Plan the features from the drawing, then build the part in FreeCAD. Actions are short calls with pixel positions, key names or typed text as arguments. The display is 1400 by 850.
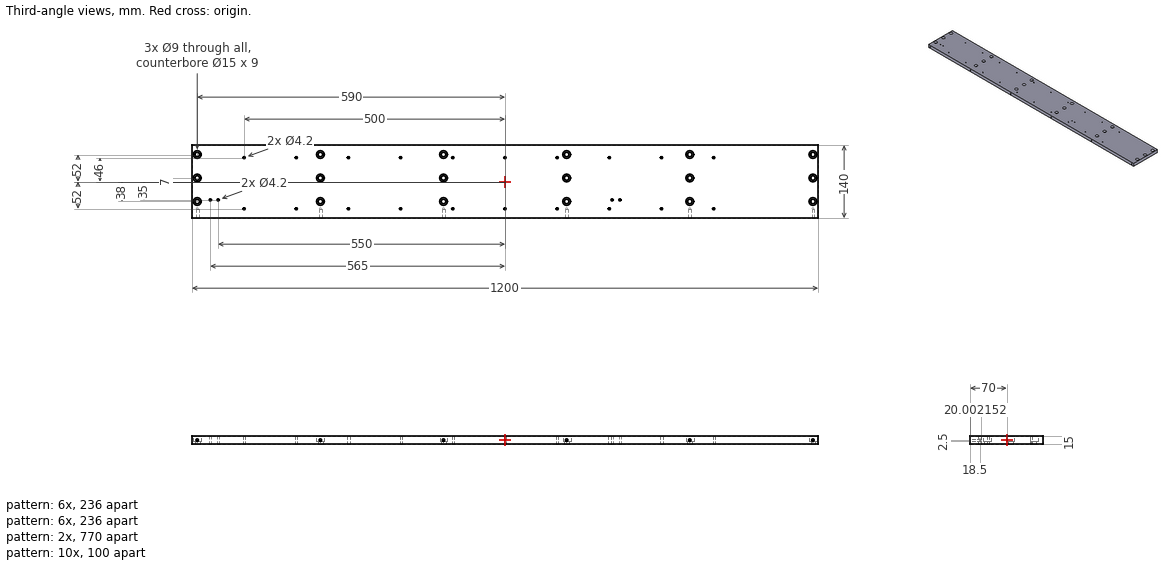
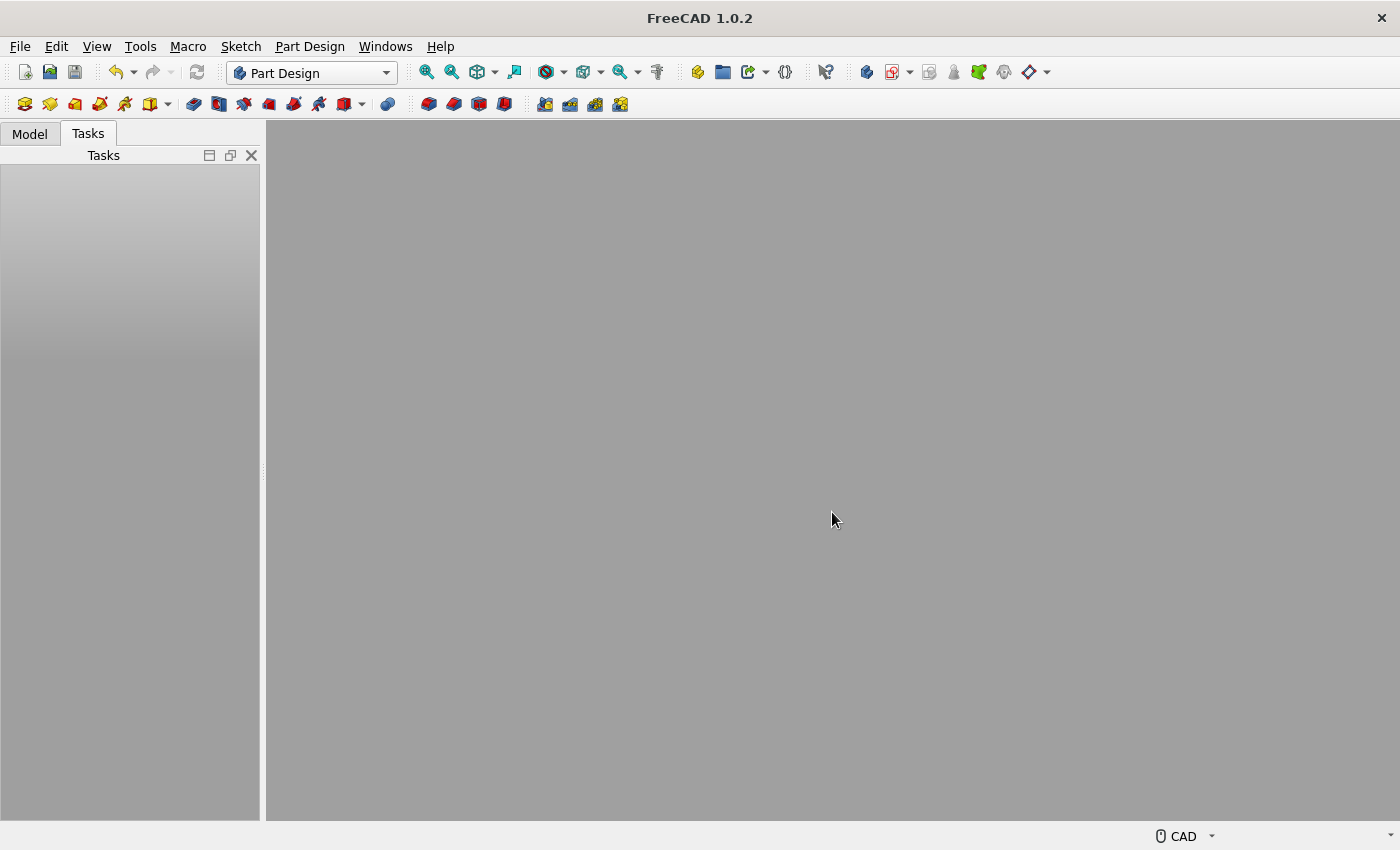
click(25, 72)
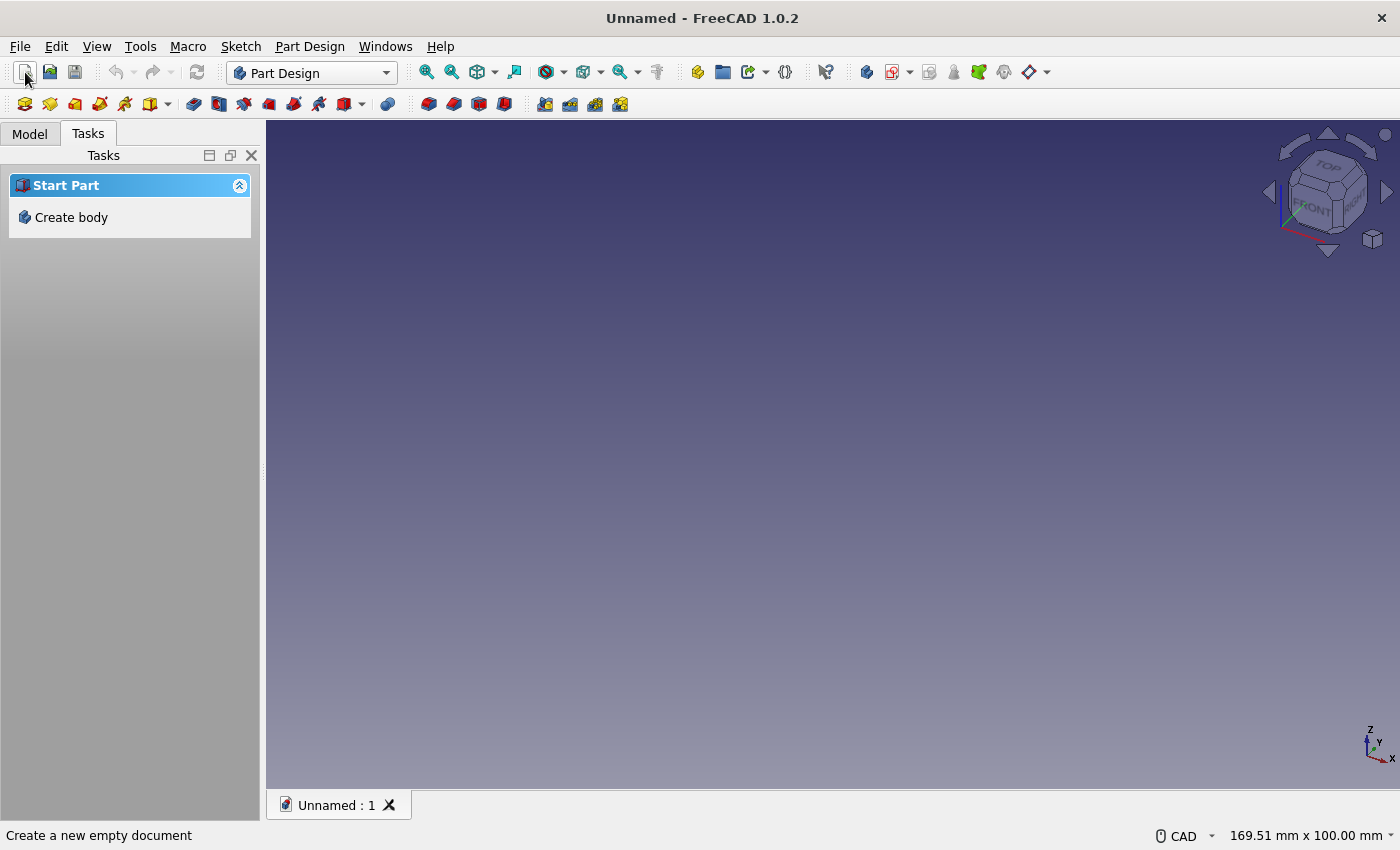
click(892, 72)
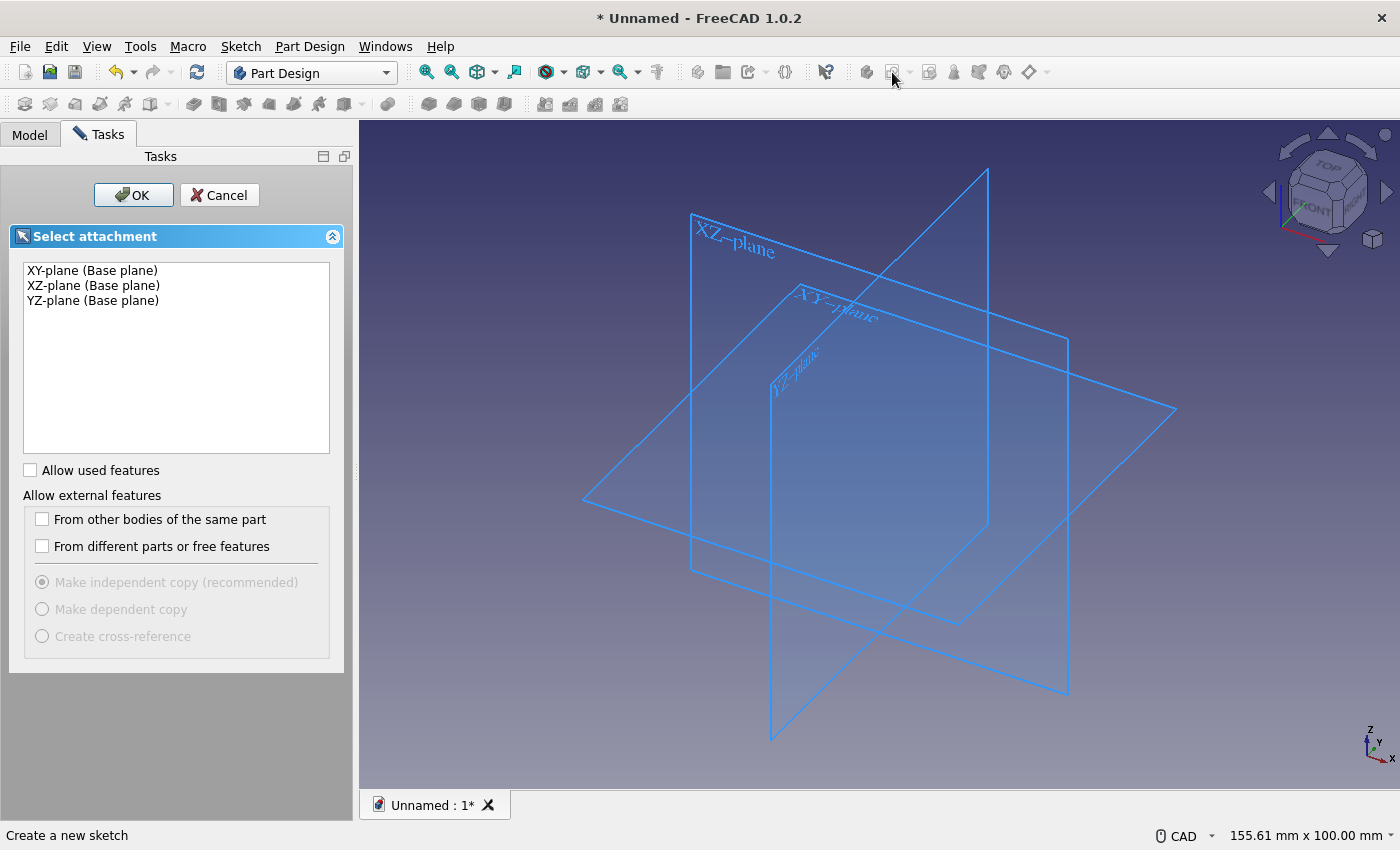
click(84, 270)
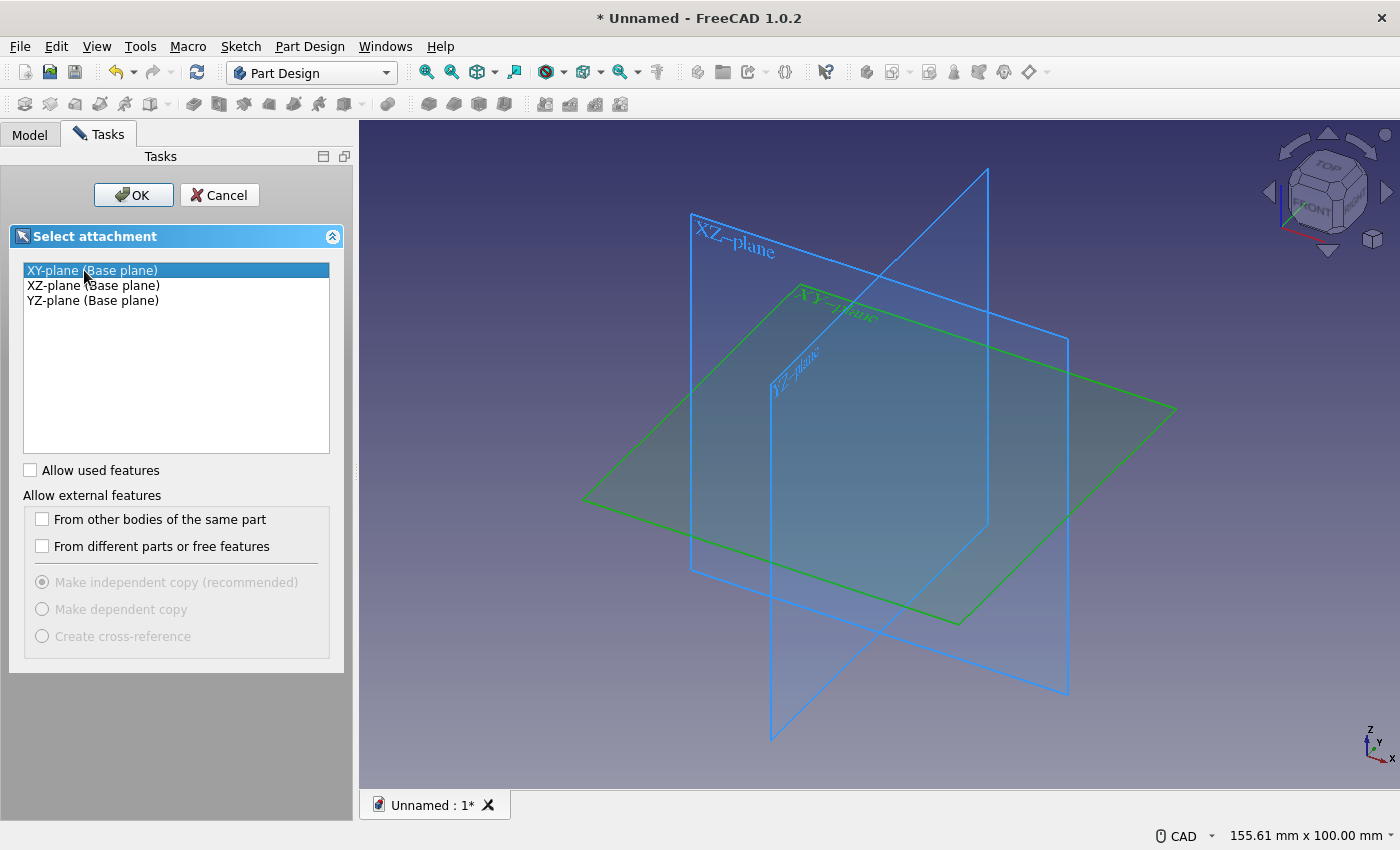
click(134, 195)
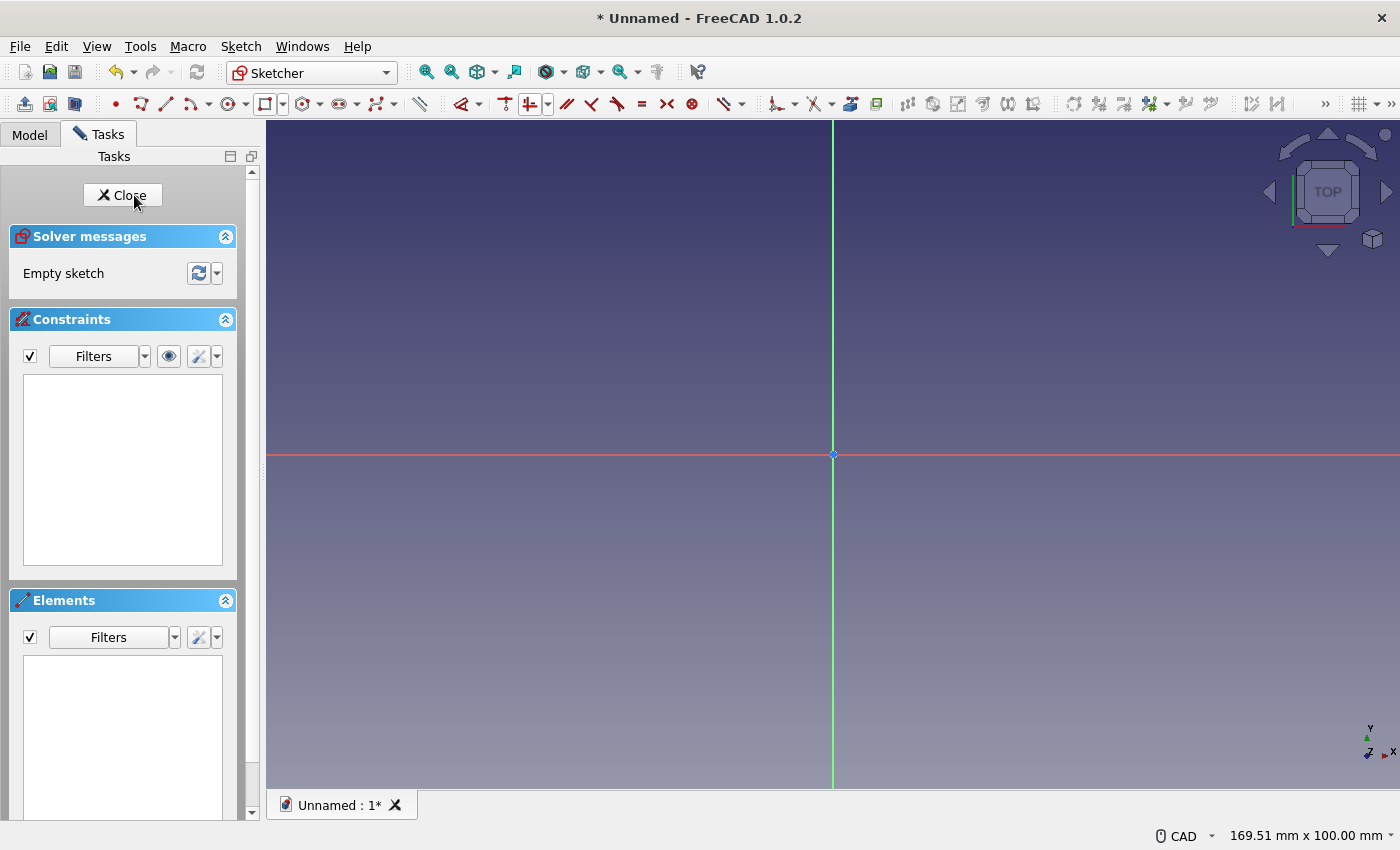
scroll(758, 454, down, 12)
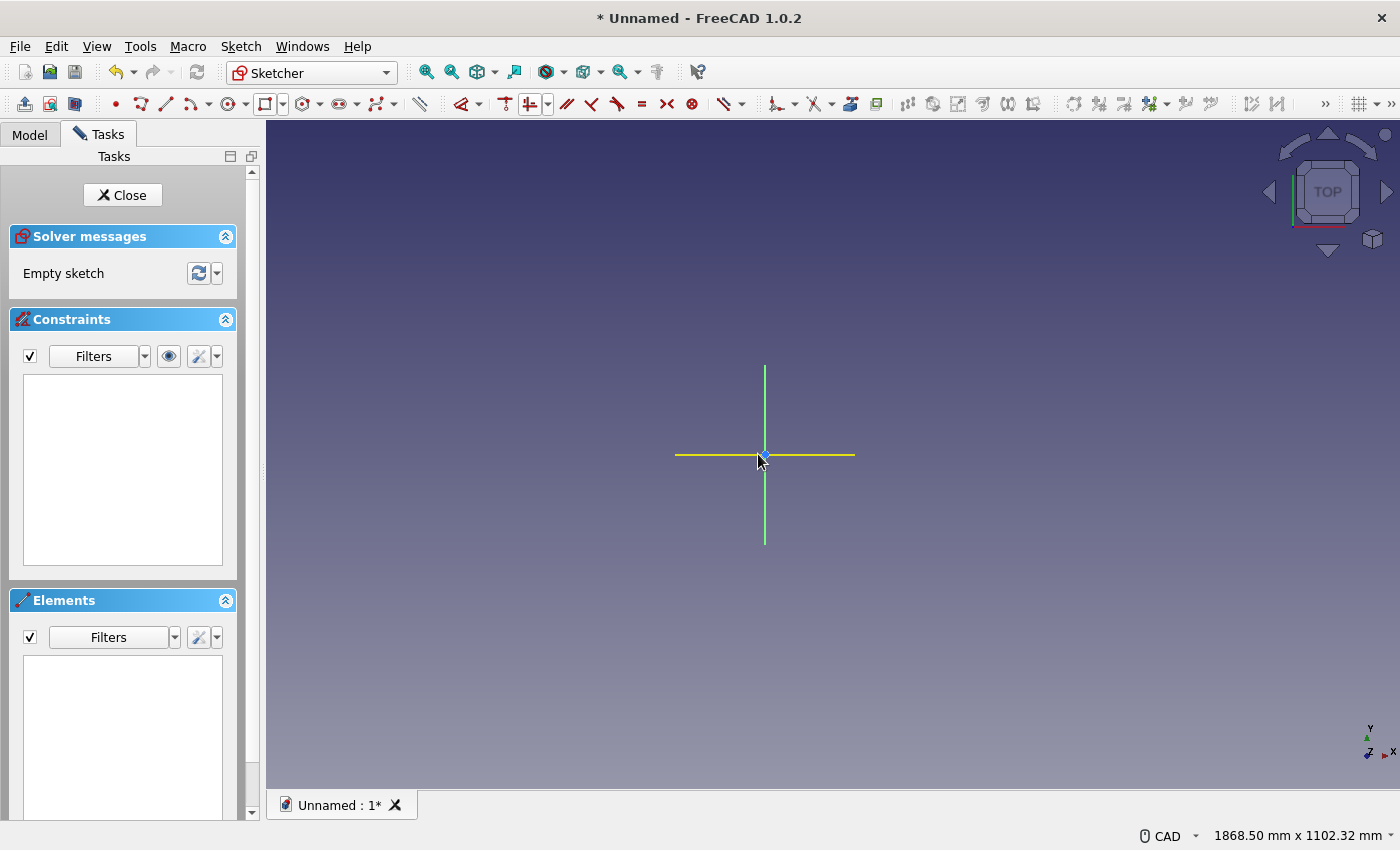
key(g)
key(v)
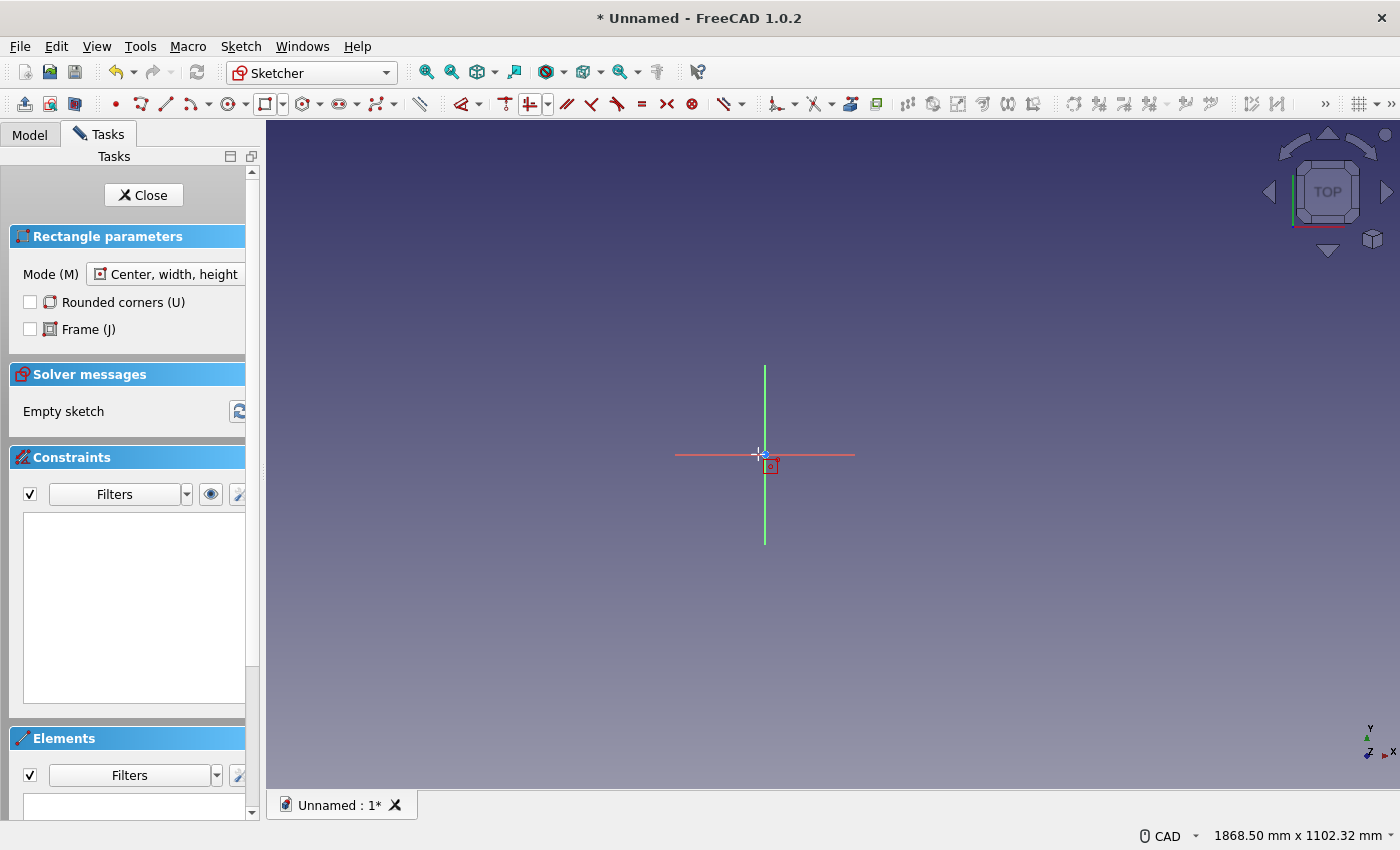
click(765, 454)
move(1129, 412)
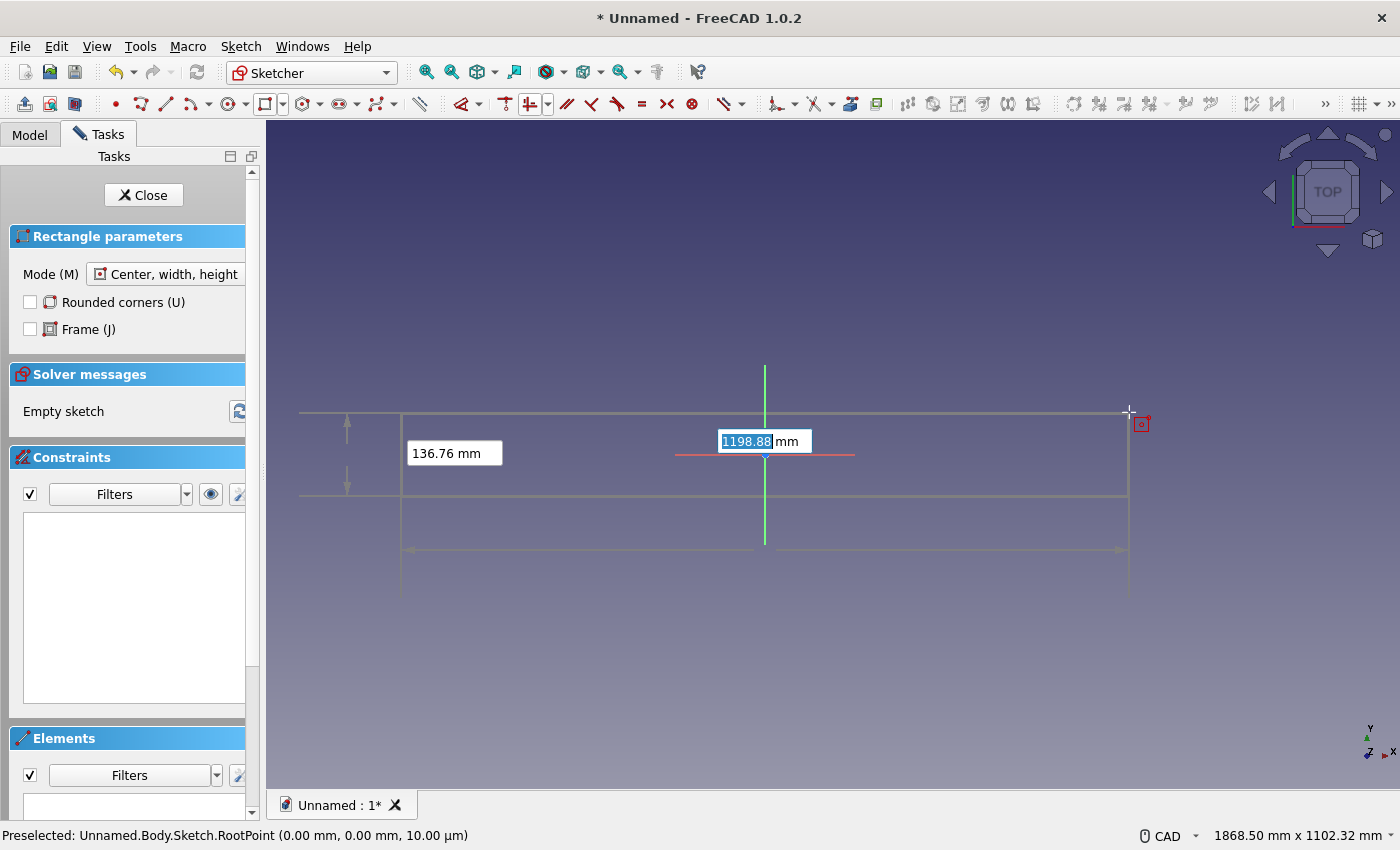
text(1200)
key(Tab)
text(140)
key(Return)
key(Escape)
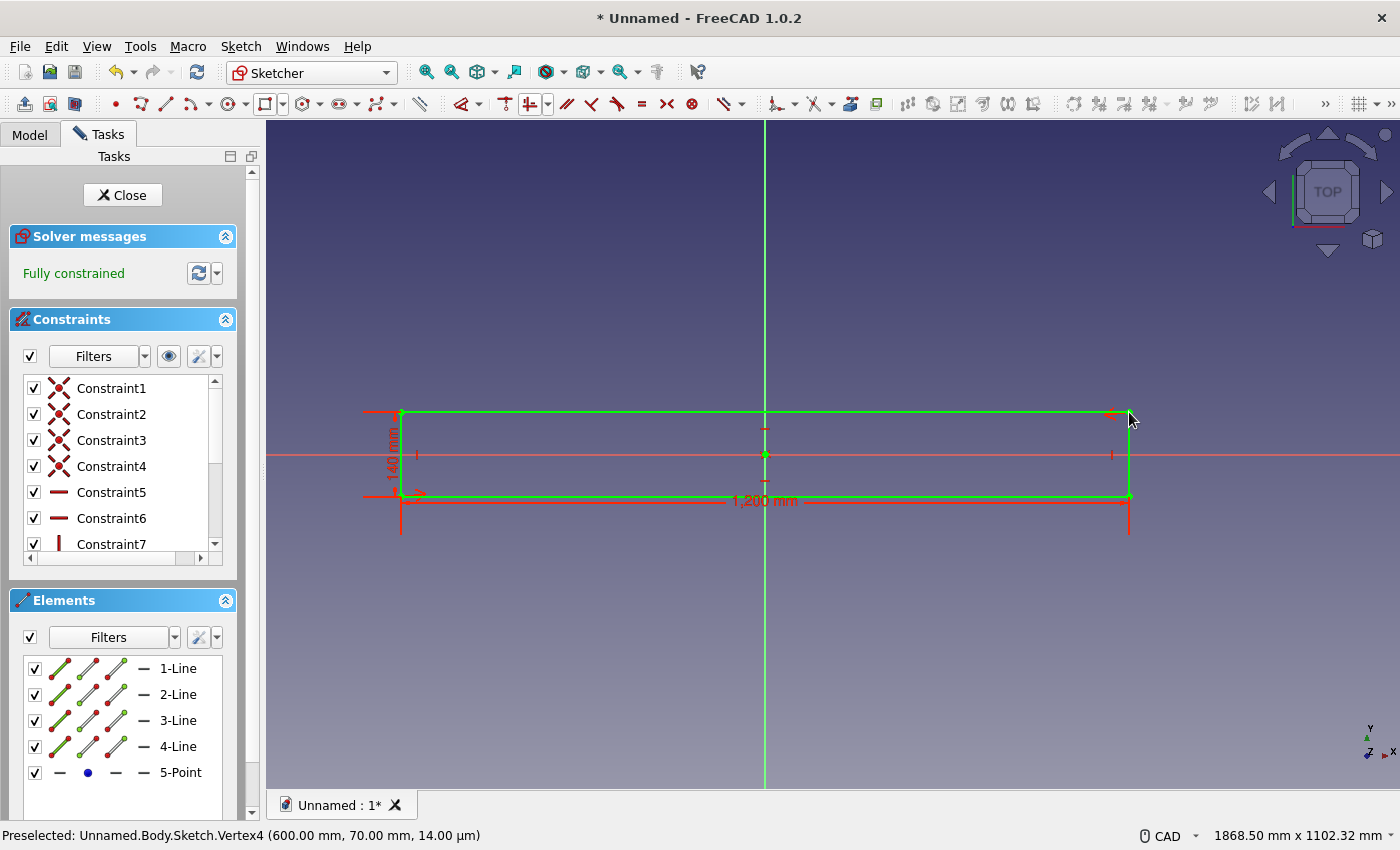
click(123, 195)